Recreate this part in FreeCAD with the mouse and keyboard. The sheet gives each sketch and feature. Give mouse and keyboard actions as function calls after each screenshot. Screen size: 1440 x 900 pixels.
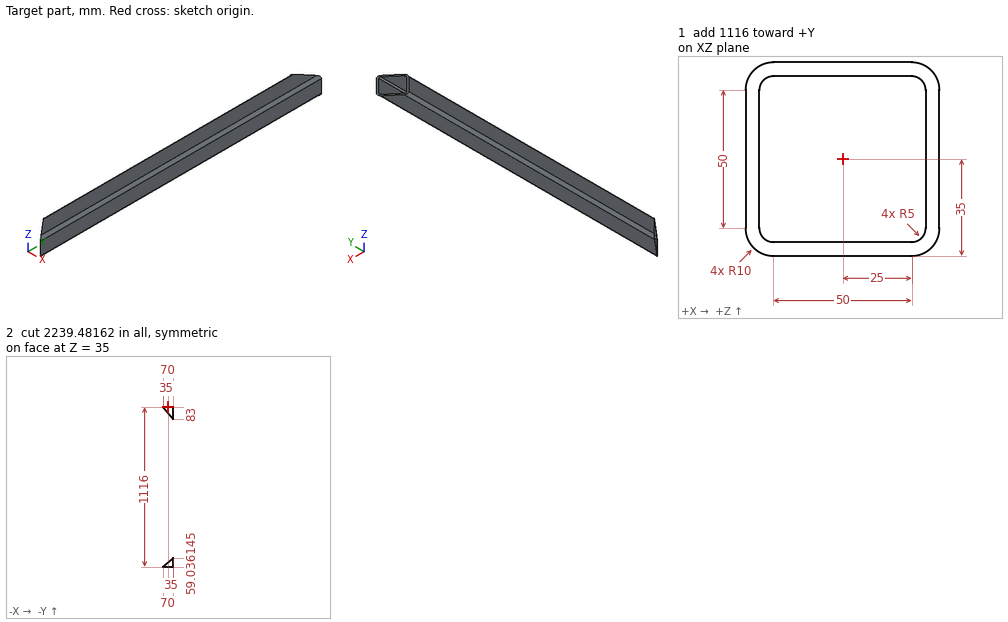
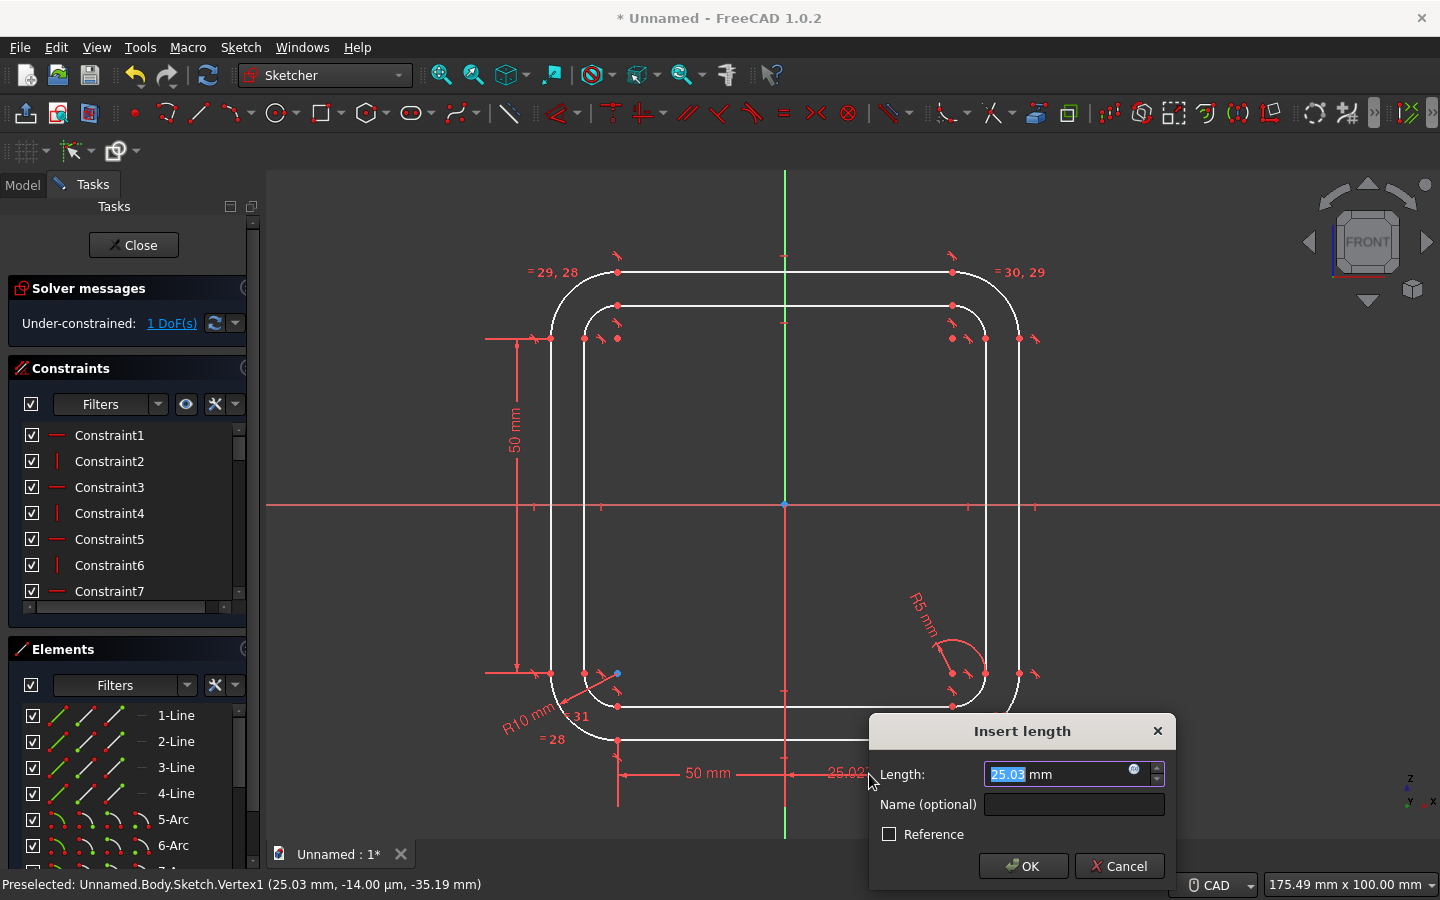
text(25)
key(Return)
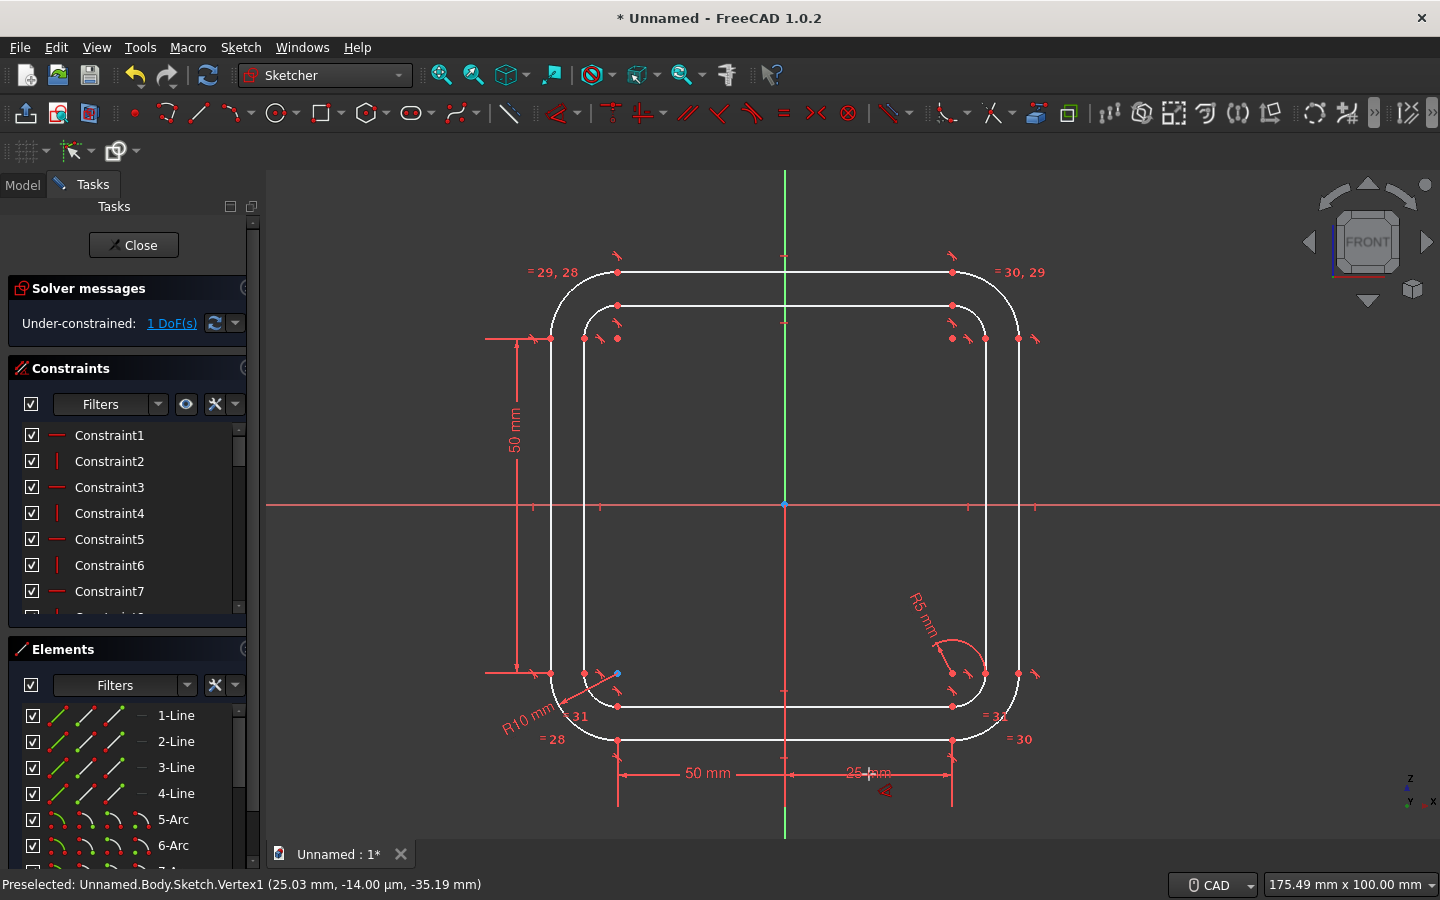
click(952, 740)
click(751, 623)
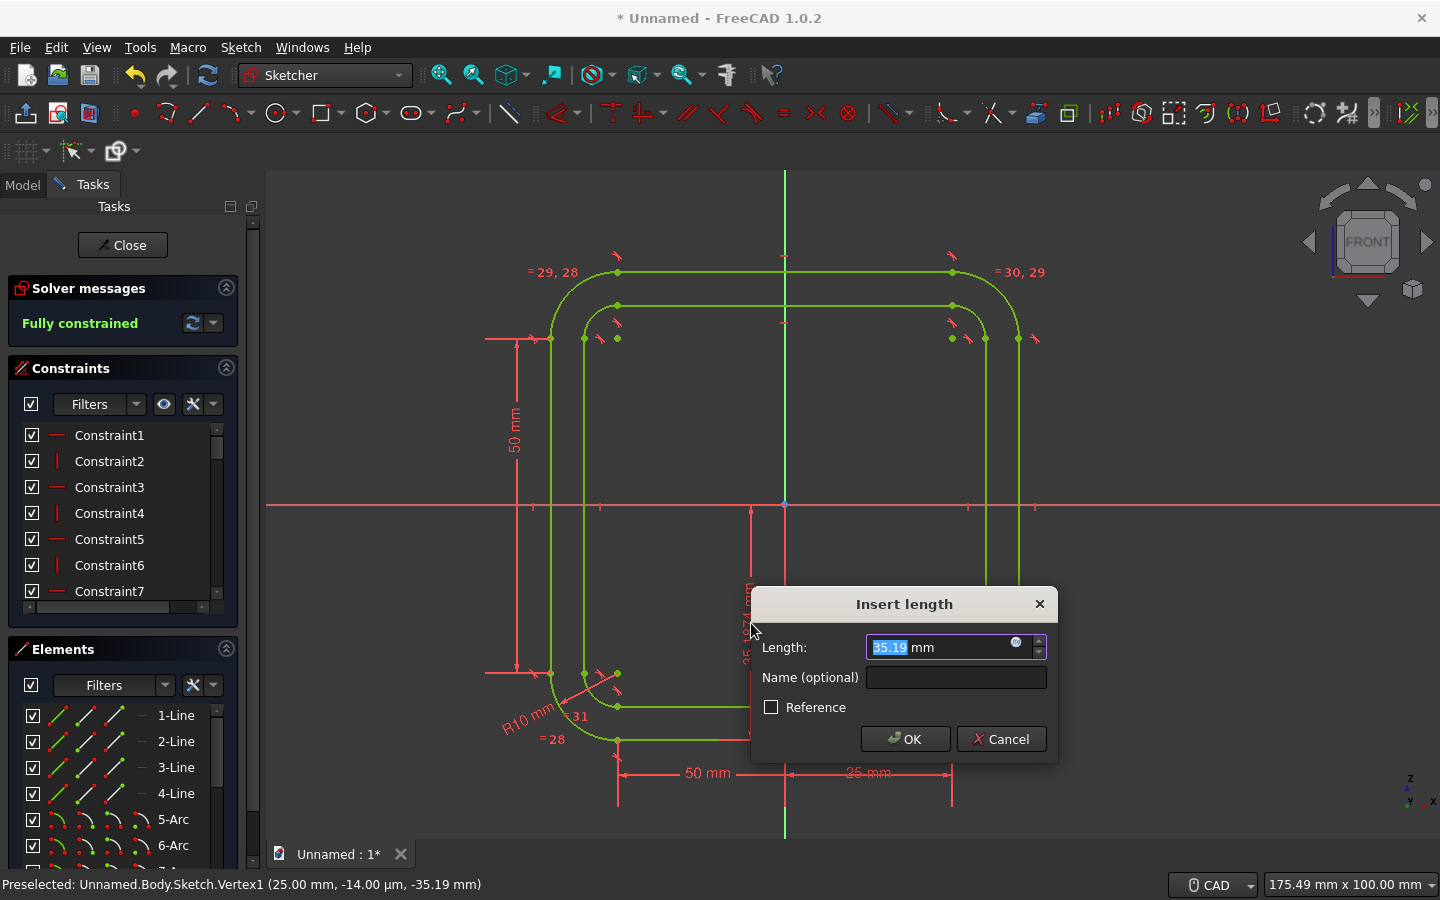
text(35)
key(Return)
key(Escape)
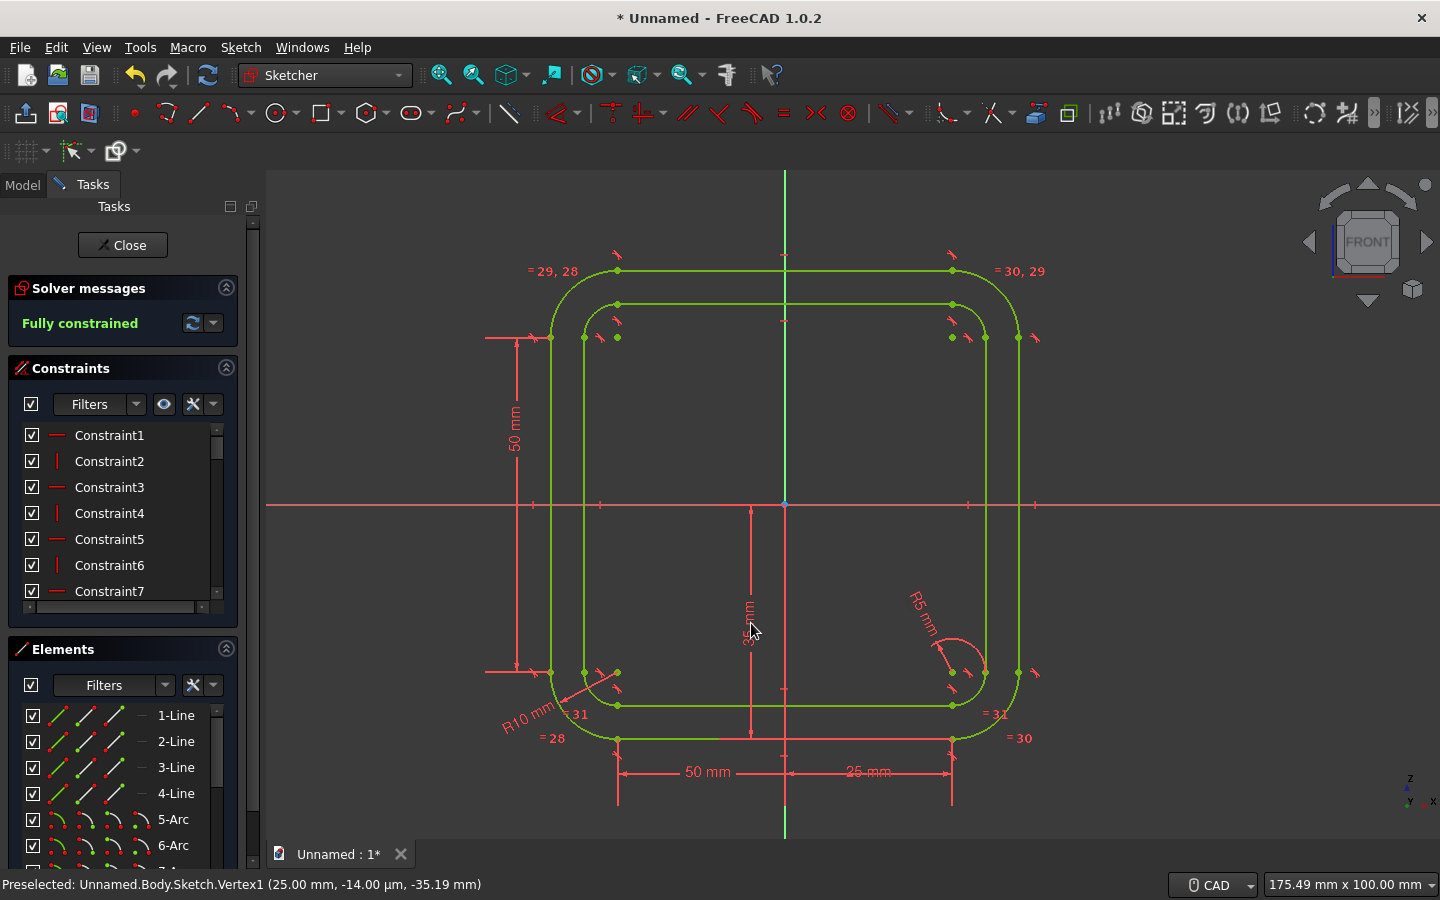
click(123, 245)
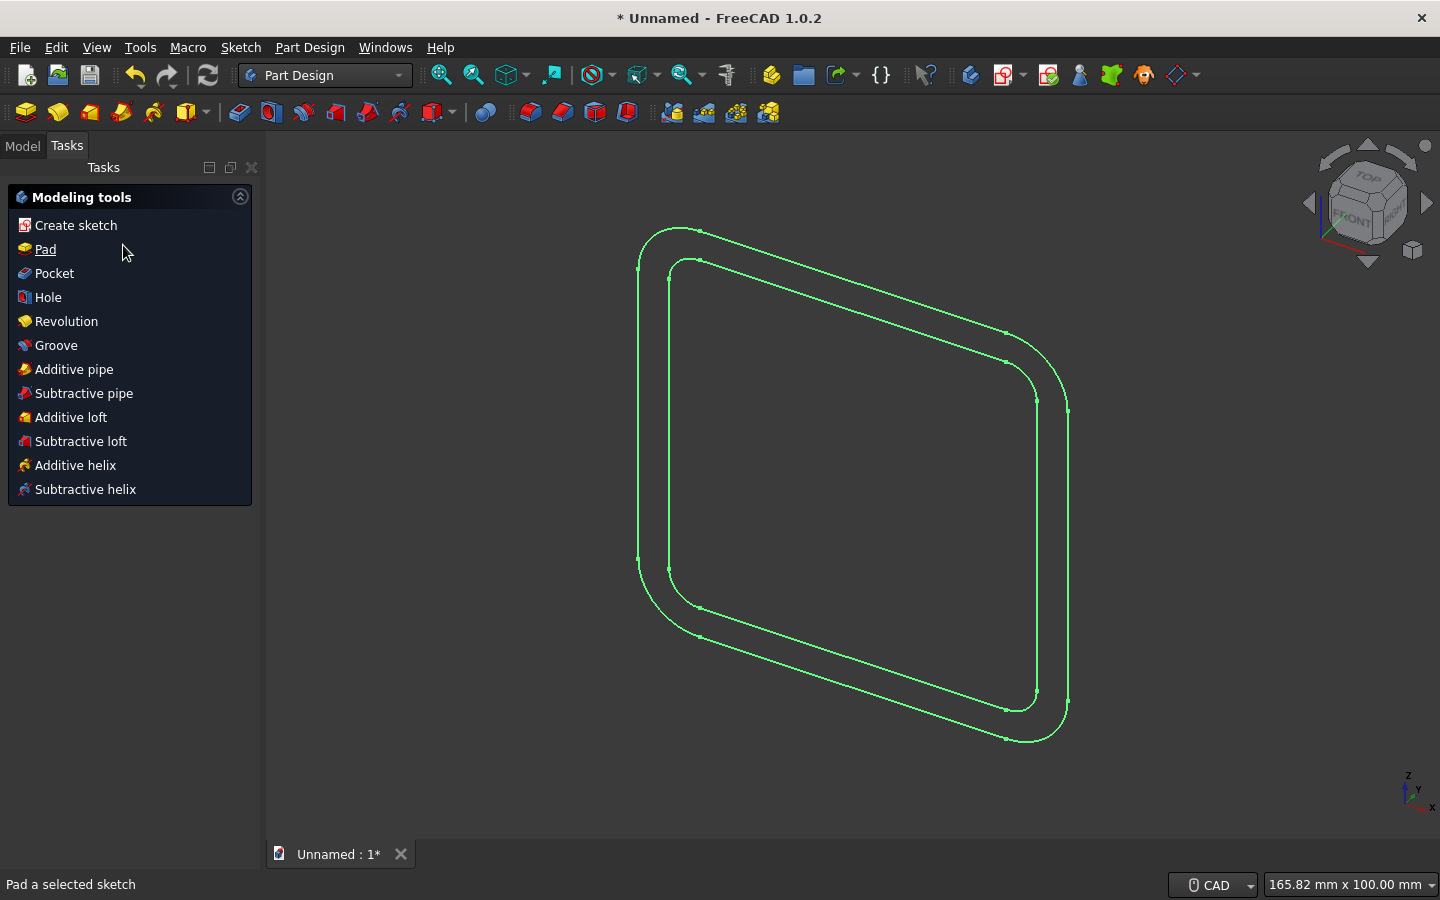
click(26, 112)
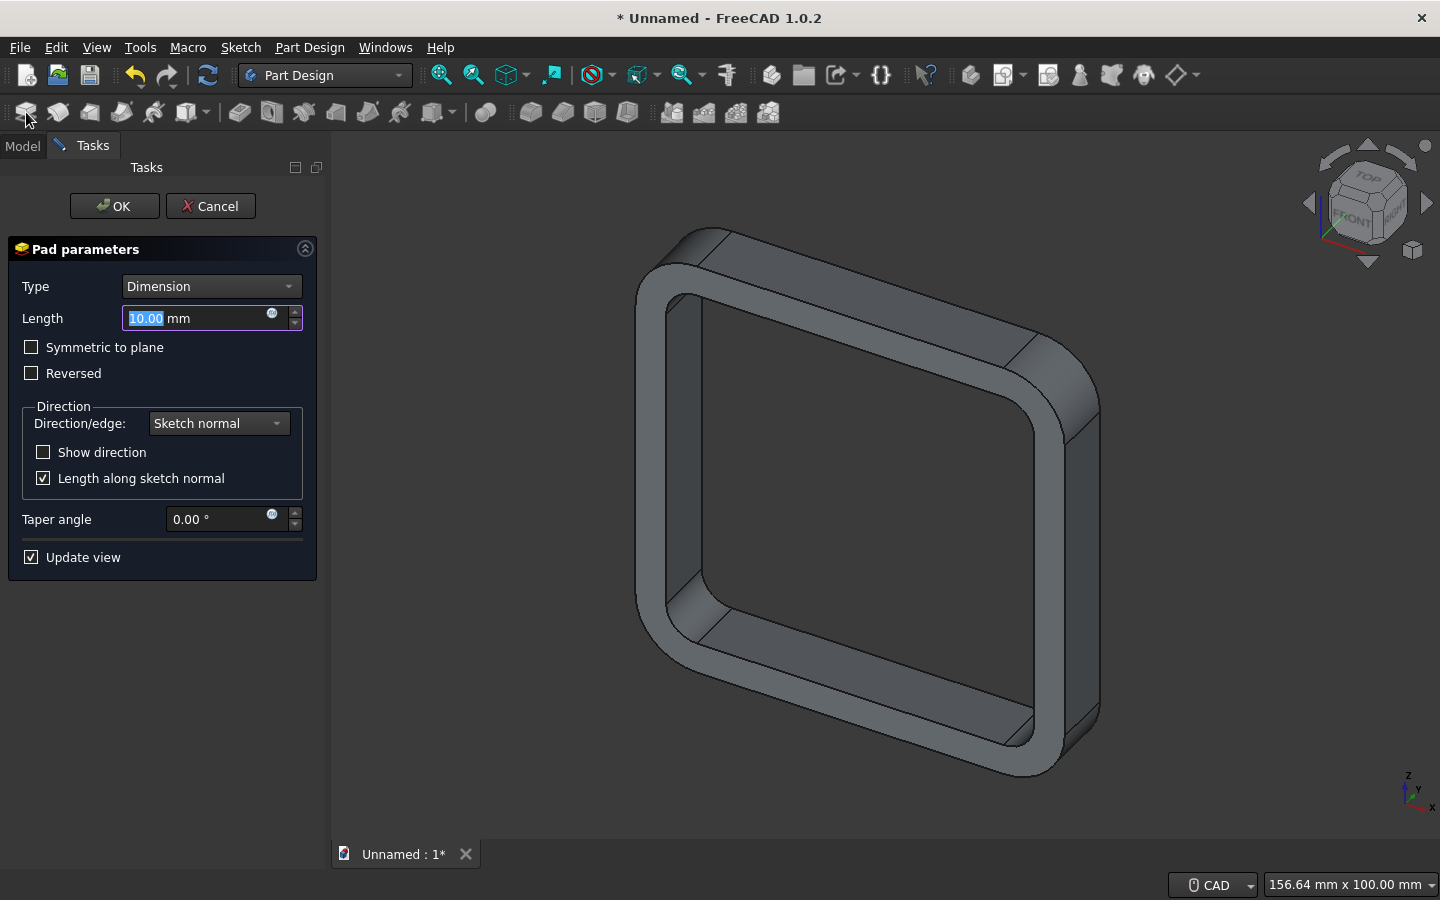
text(1116)
key(Tab)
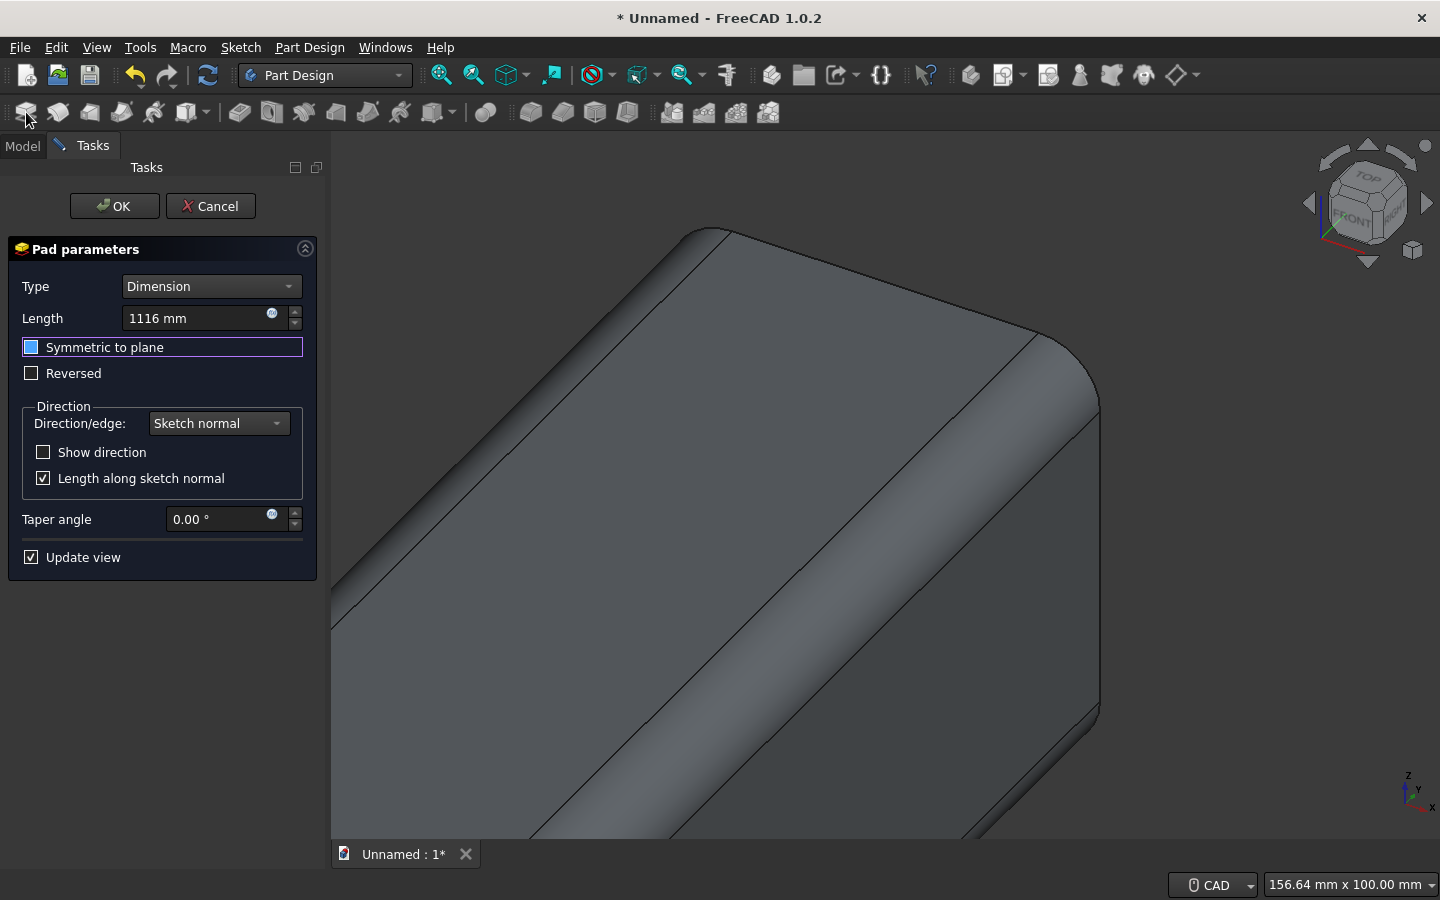
click(30, 373)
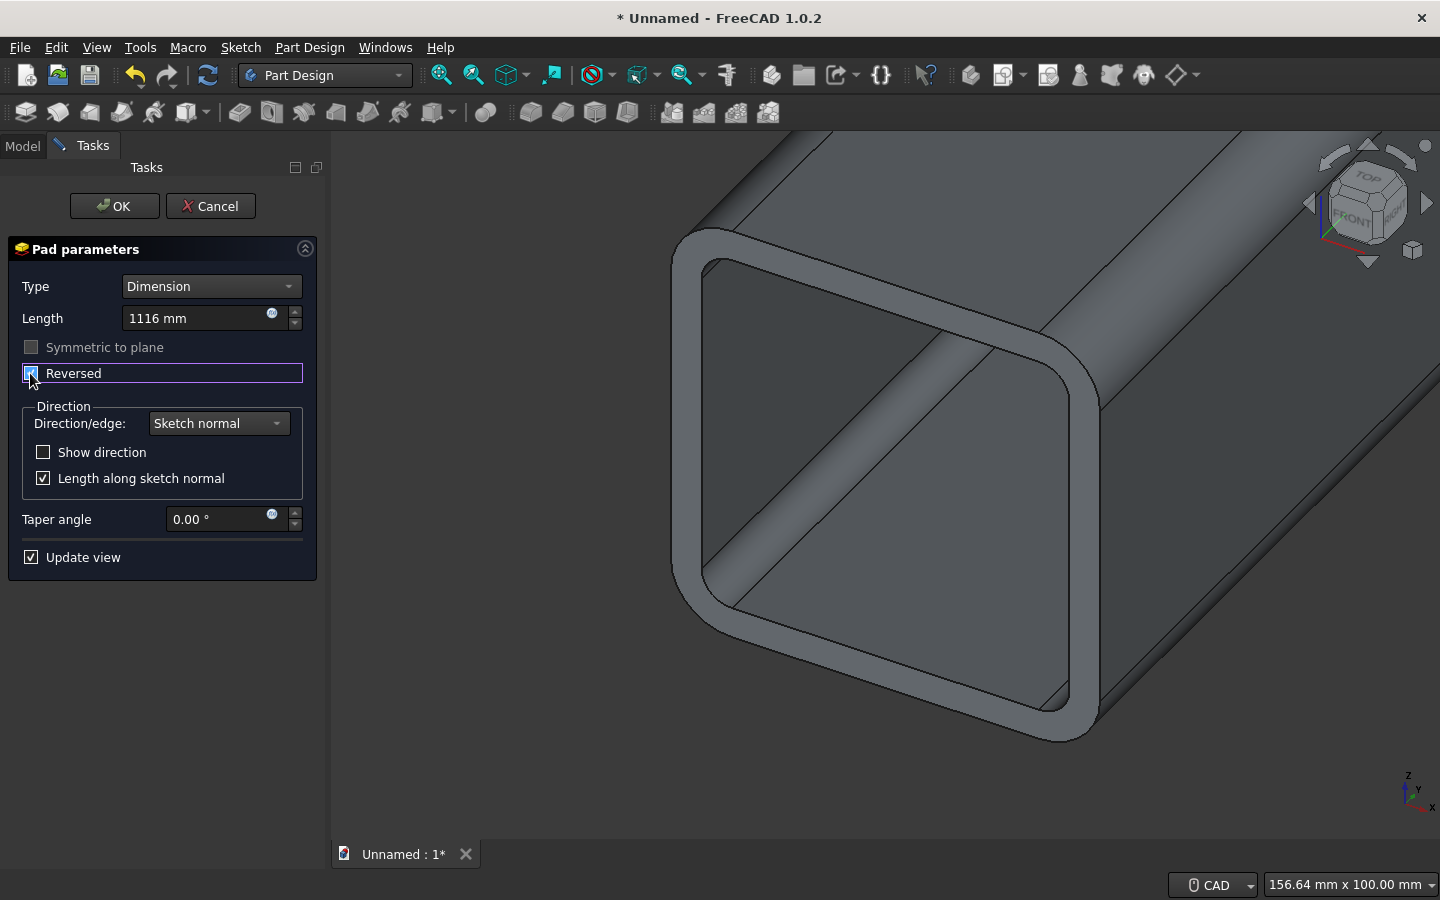
click(115, 206)